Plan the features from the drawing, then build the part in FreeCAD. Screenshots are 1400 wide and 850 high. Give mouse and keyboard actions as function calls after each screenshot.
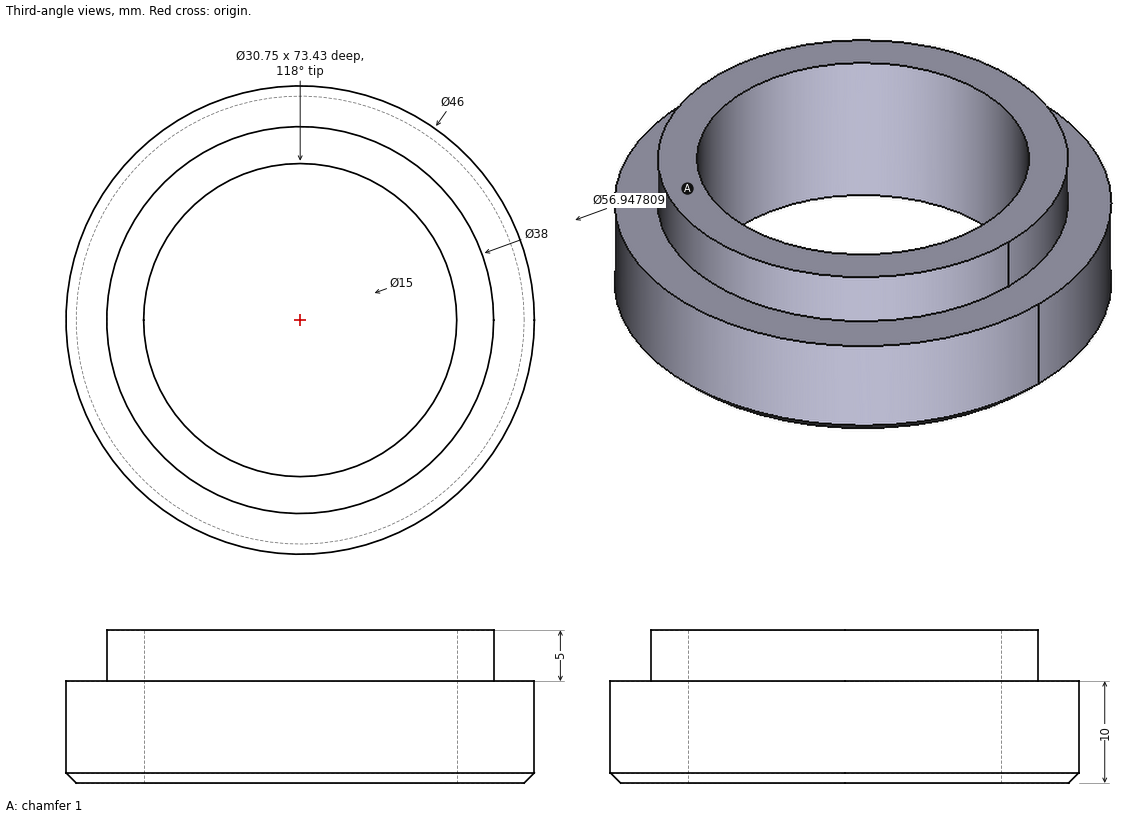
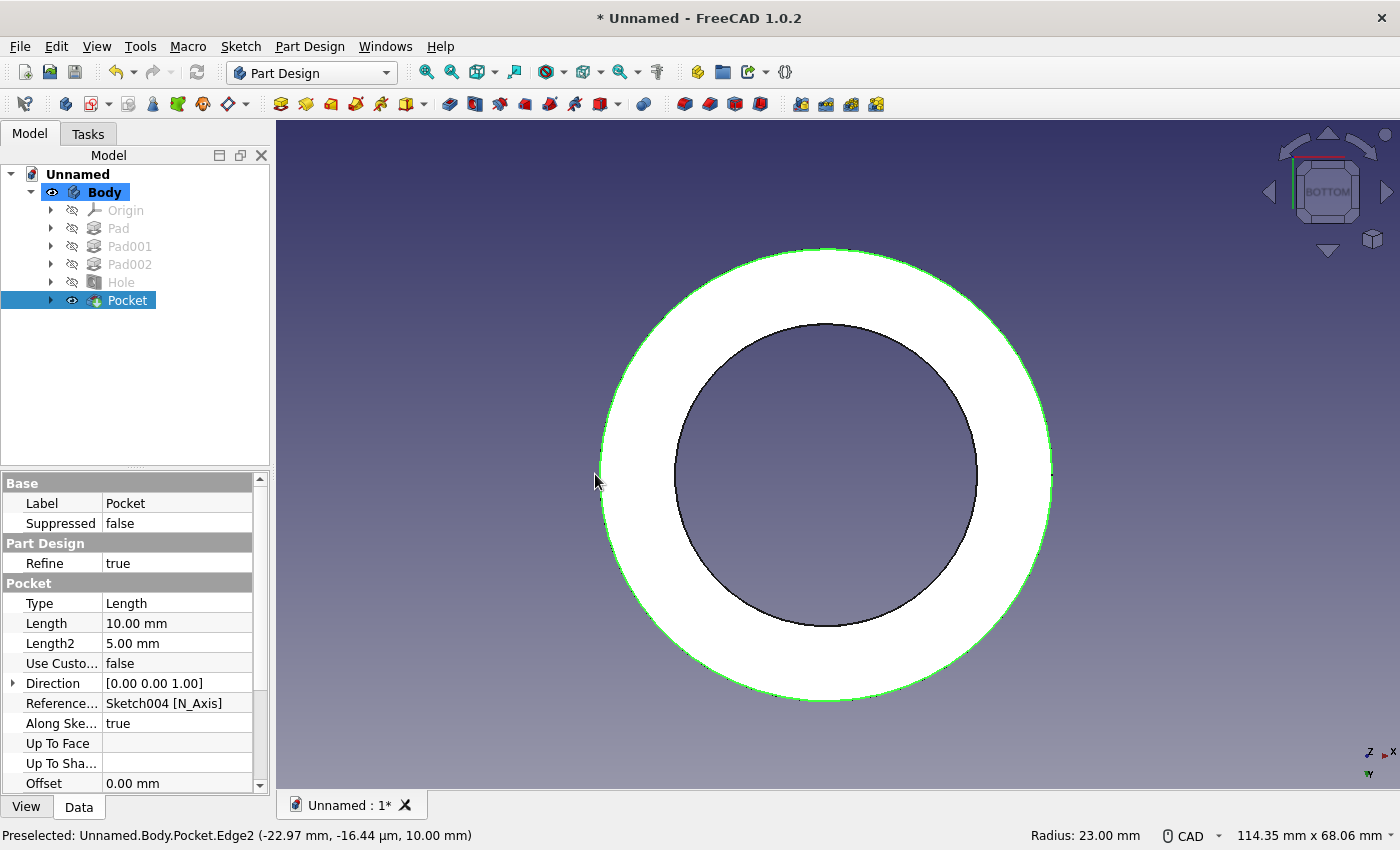
click(710, 104)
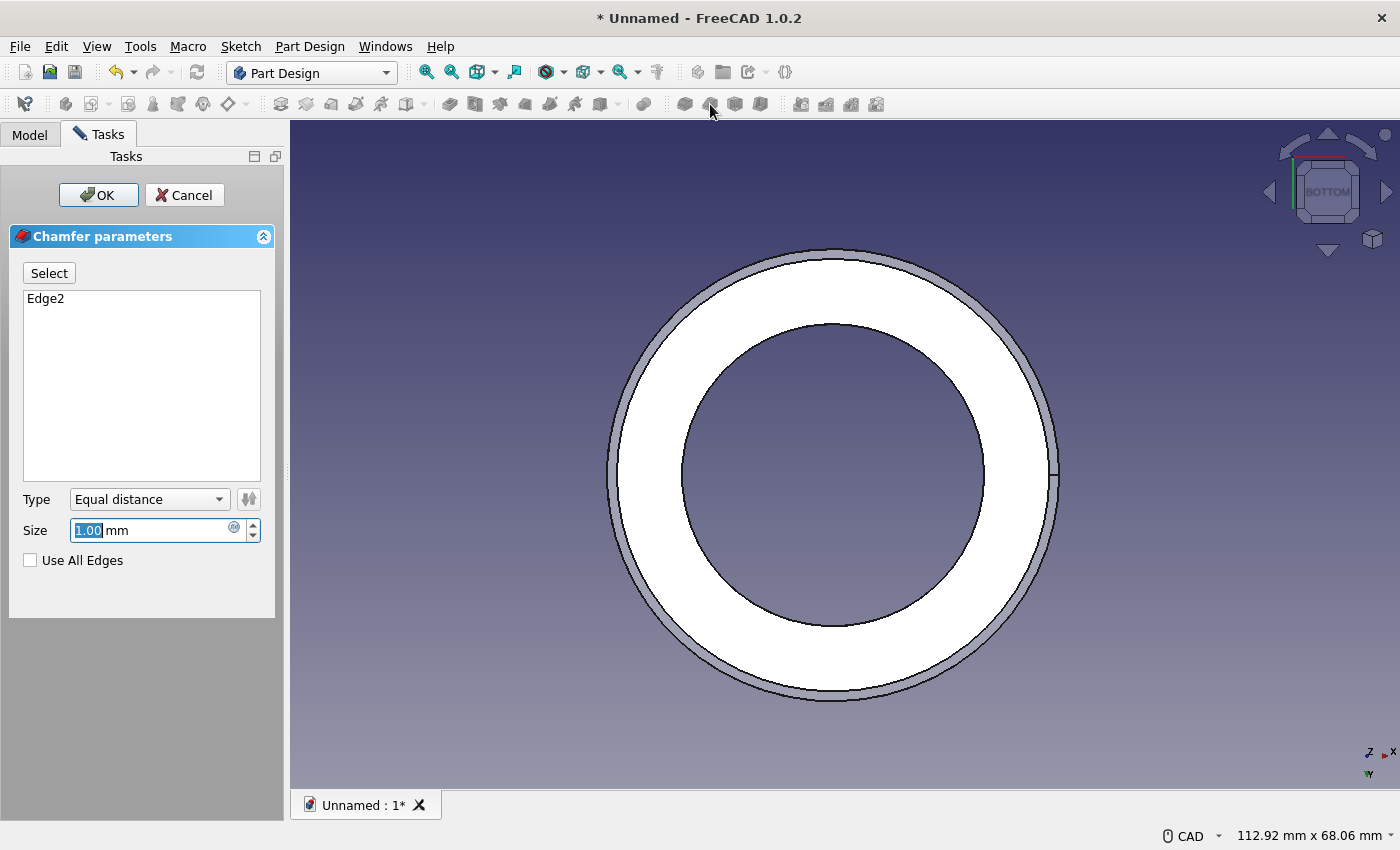
text(1)
key(Tab)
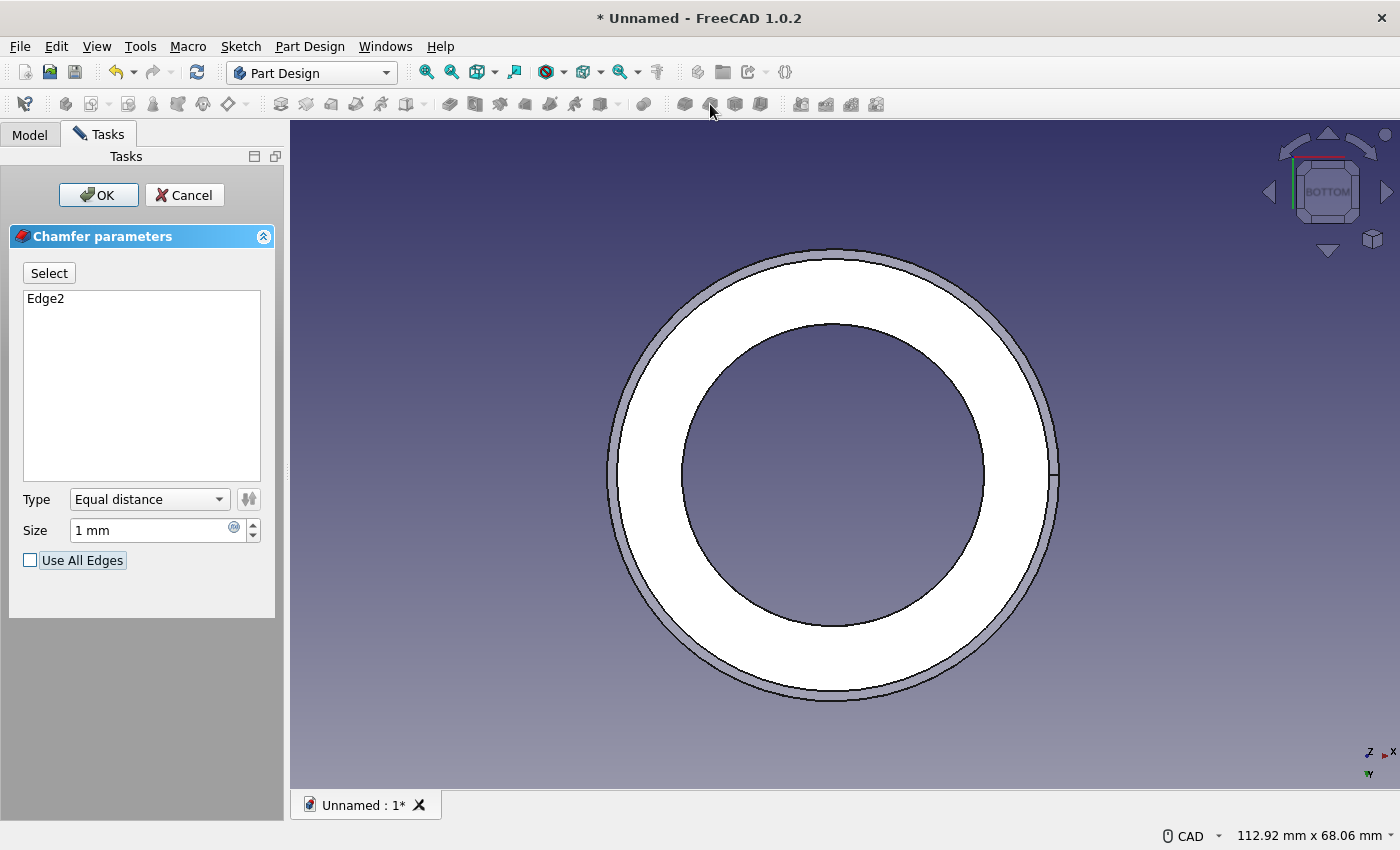
click(99, 195)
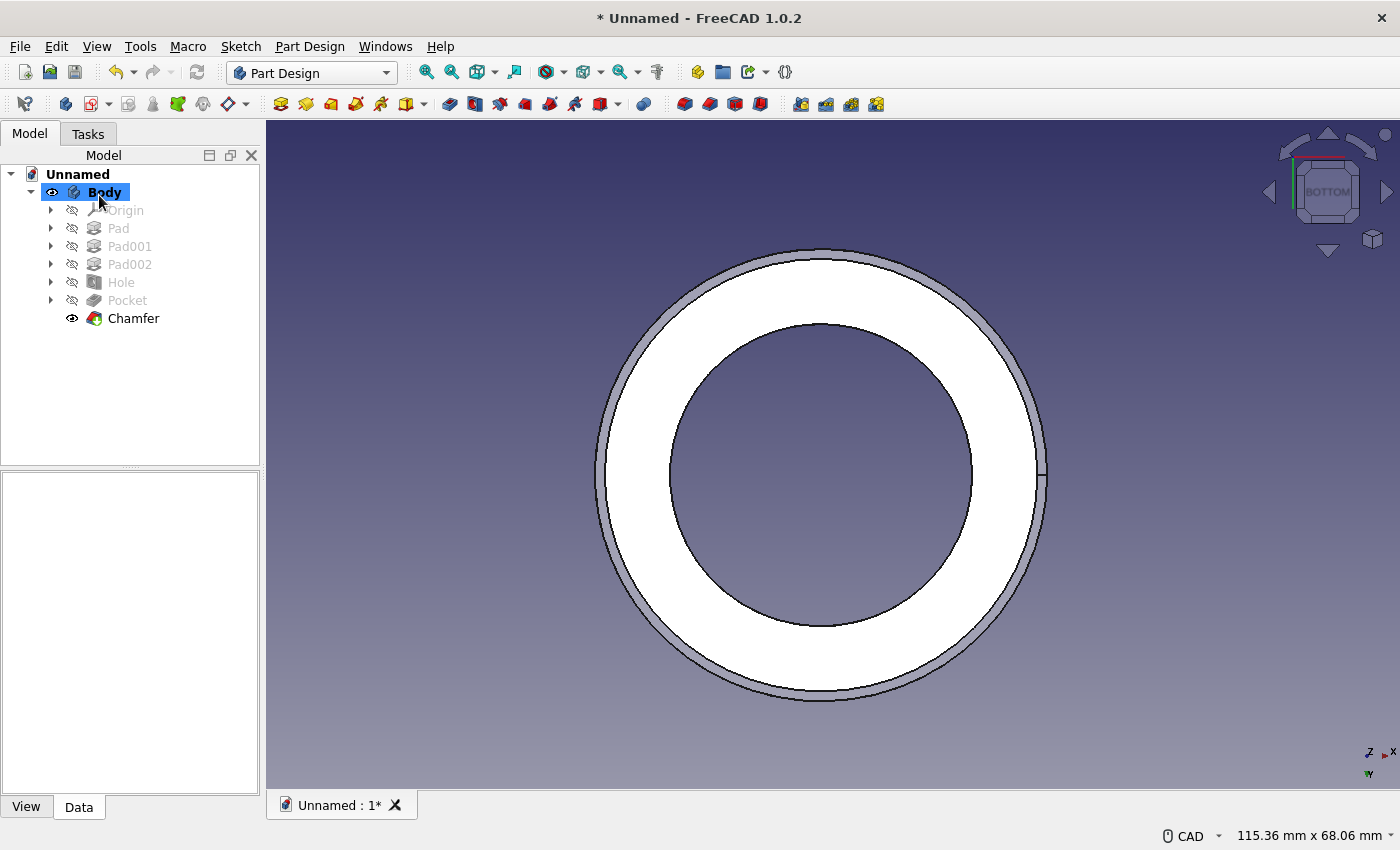
key(0)